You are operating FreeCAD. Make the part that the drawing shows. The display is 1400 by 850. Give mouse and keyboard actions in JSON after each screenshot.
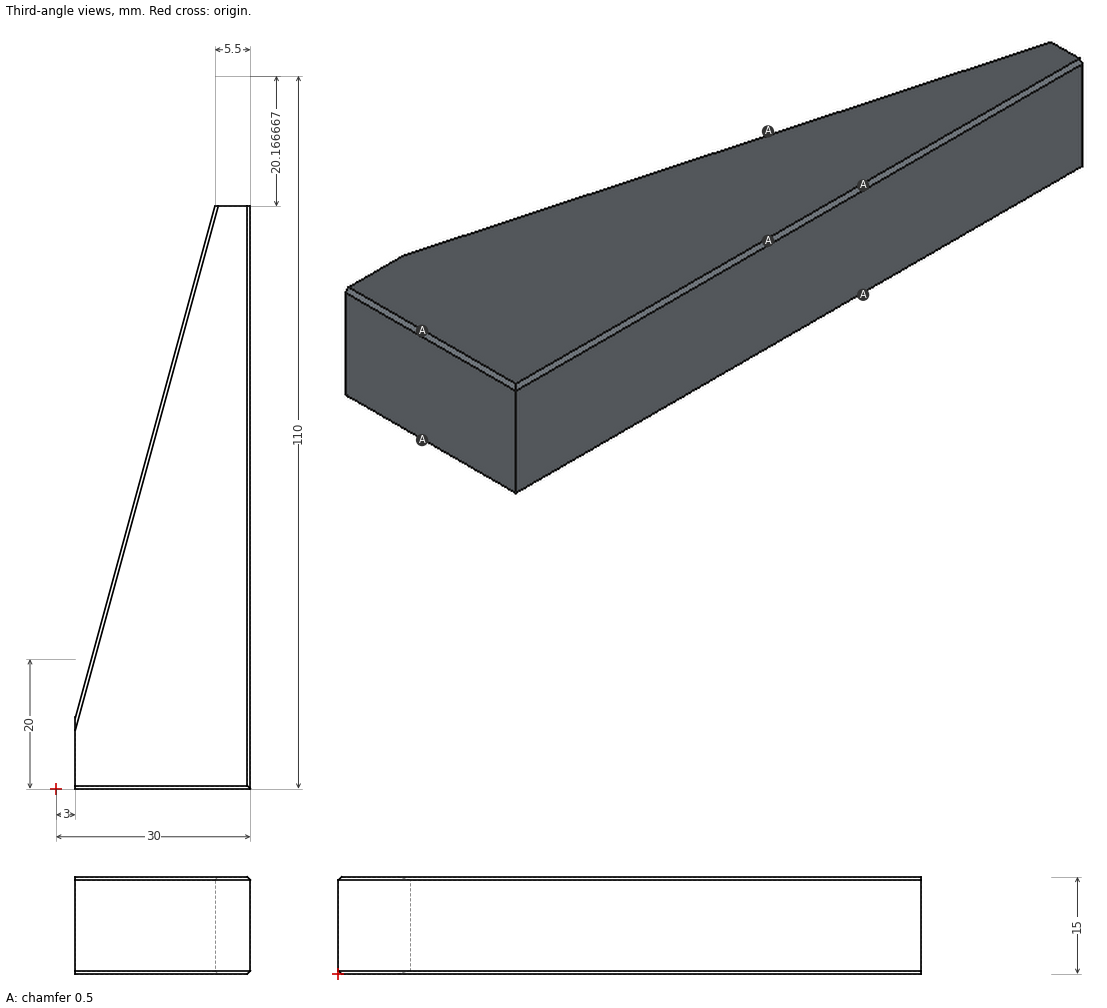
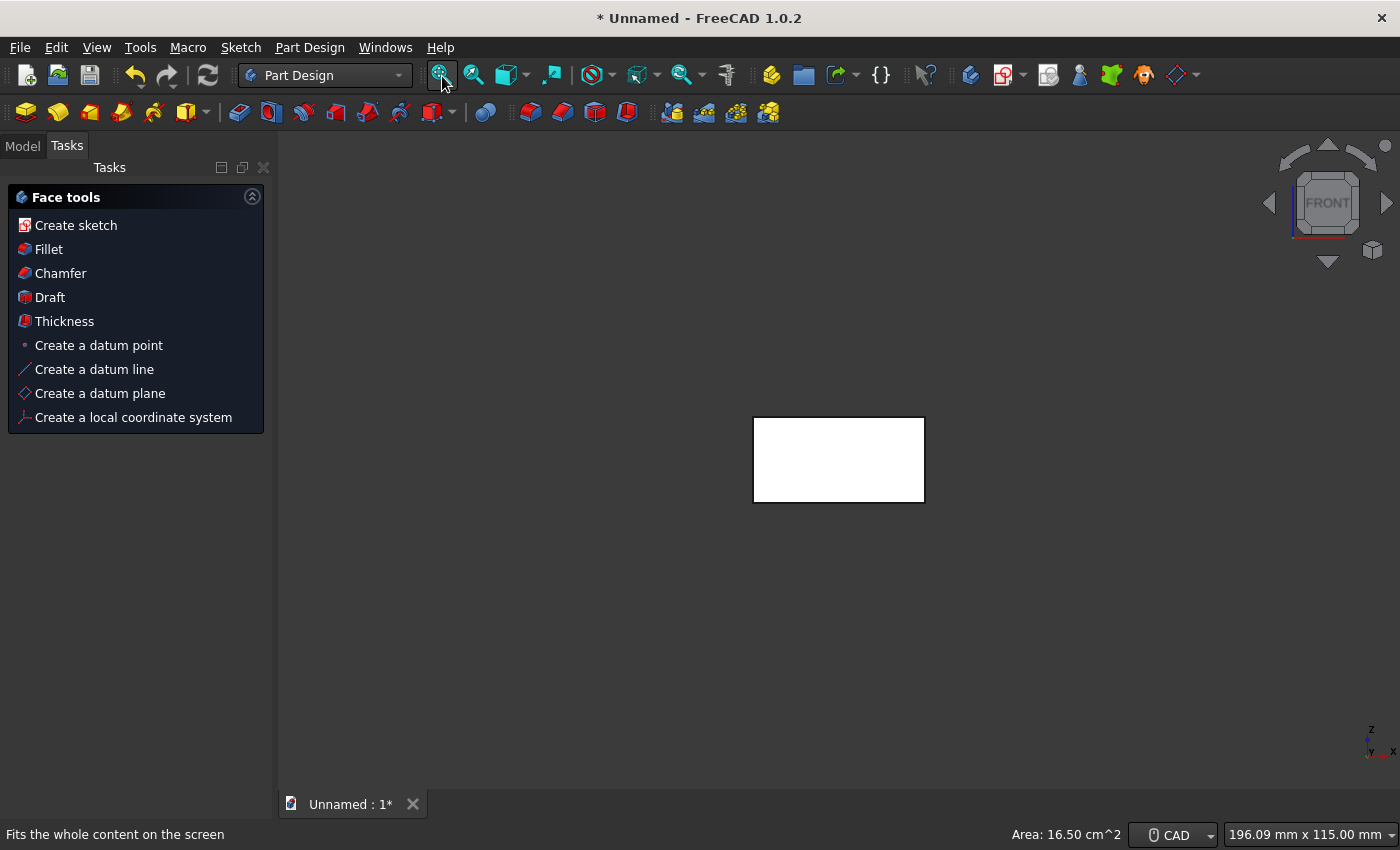
{"action": "key", "text": "3"}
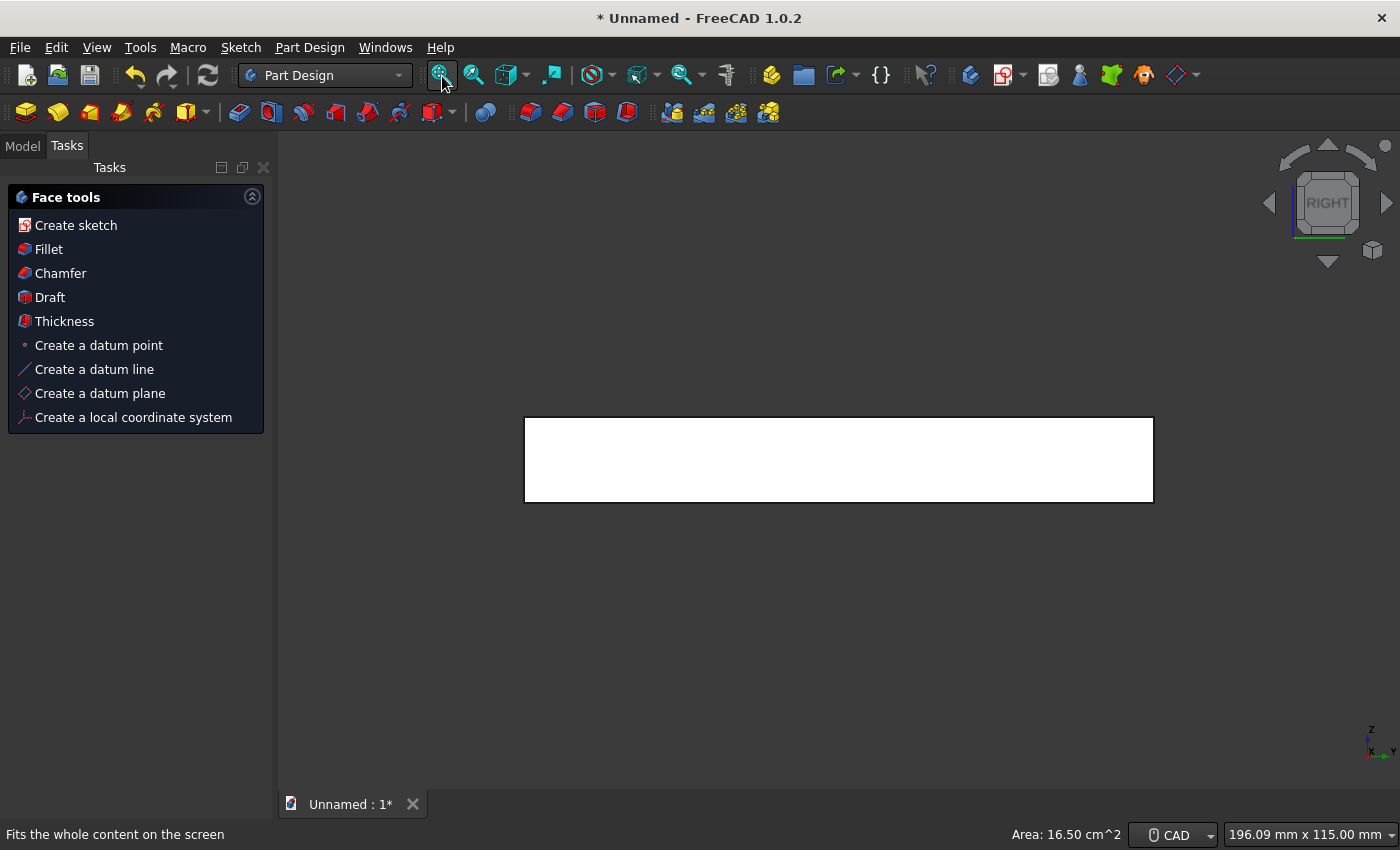
{"action": "key", "text": "5"}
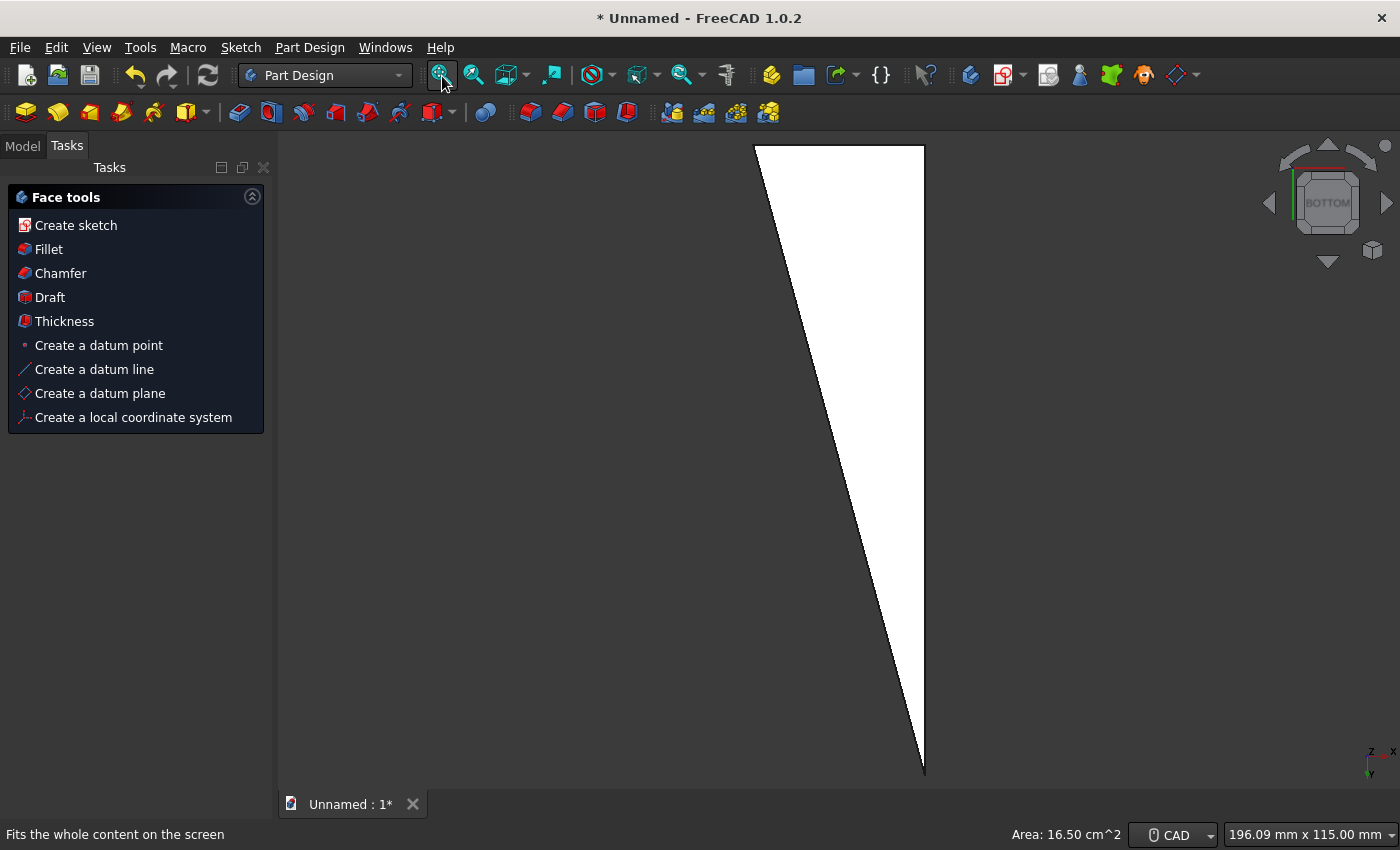
{"action": "left_click", "coordinate": [864, 279], "text": "ctrl"}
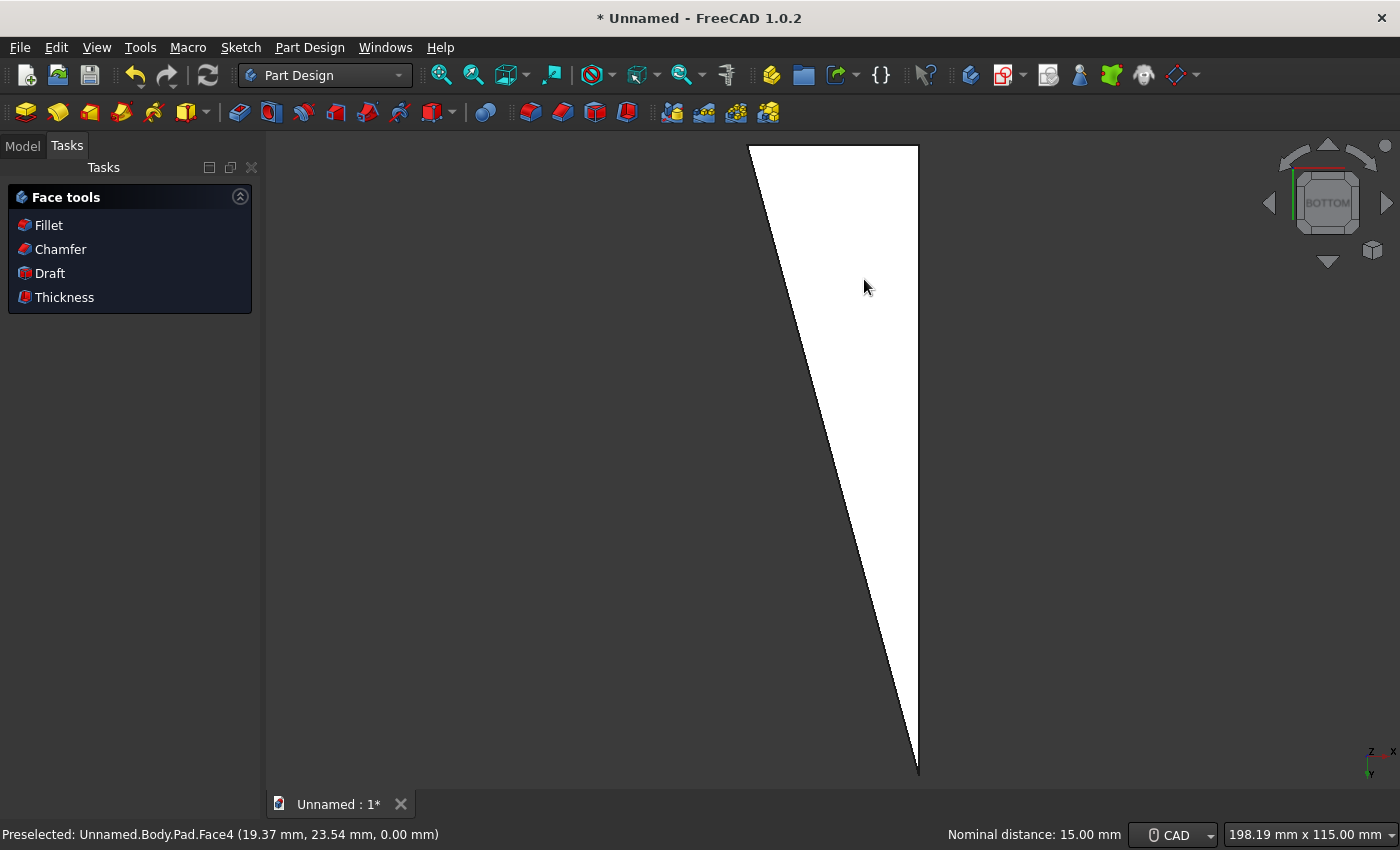
{"action": "left_click", "coordinate": [564, 112]}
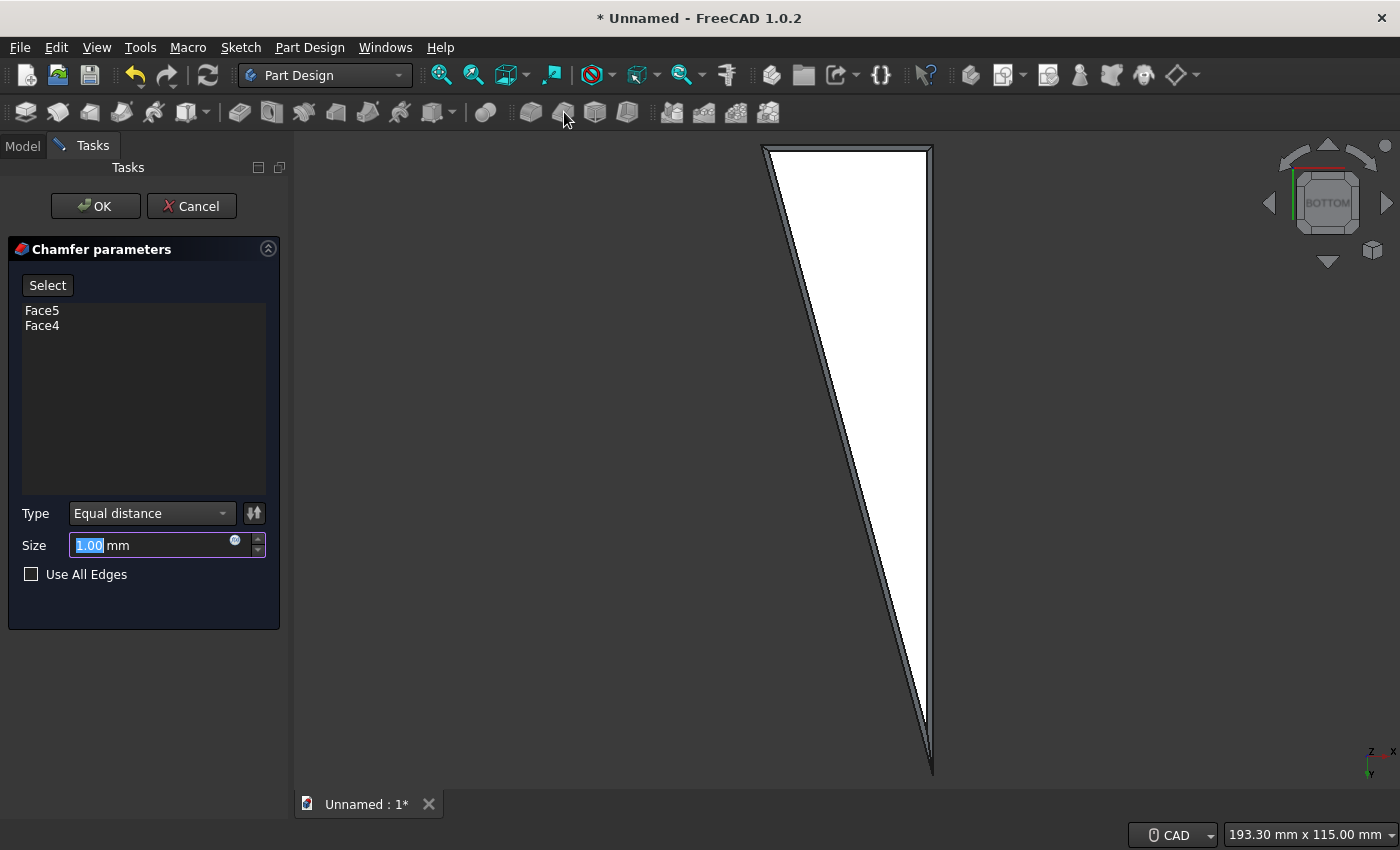
{"action": "type", "text": "0.5"}
{"action": "key", "text": "Tab"}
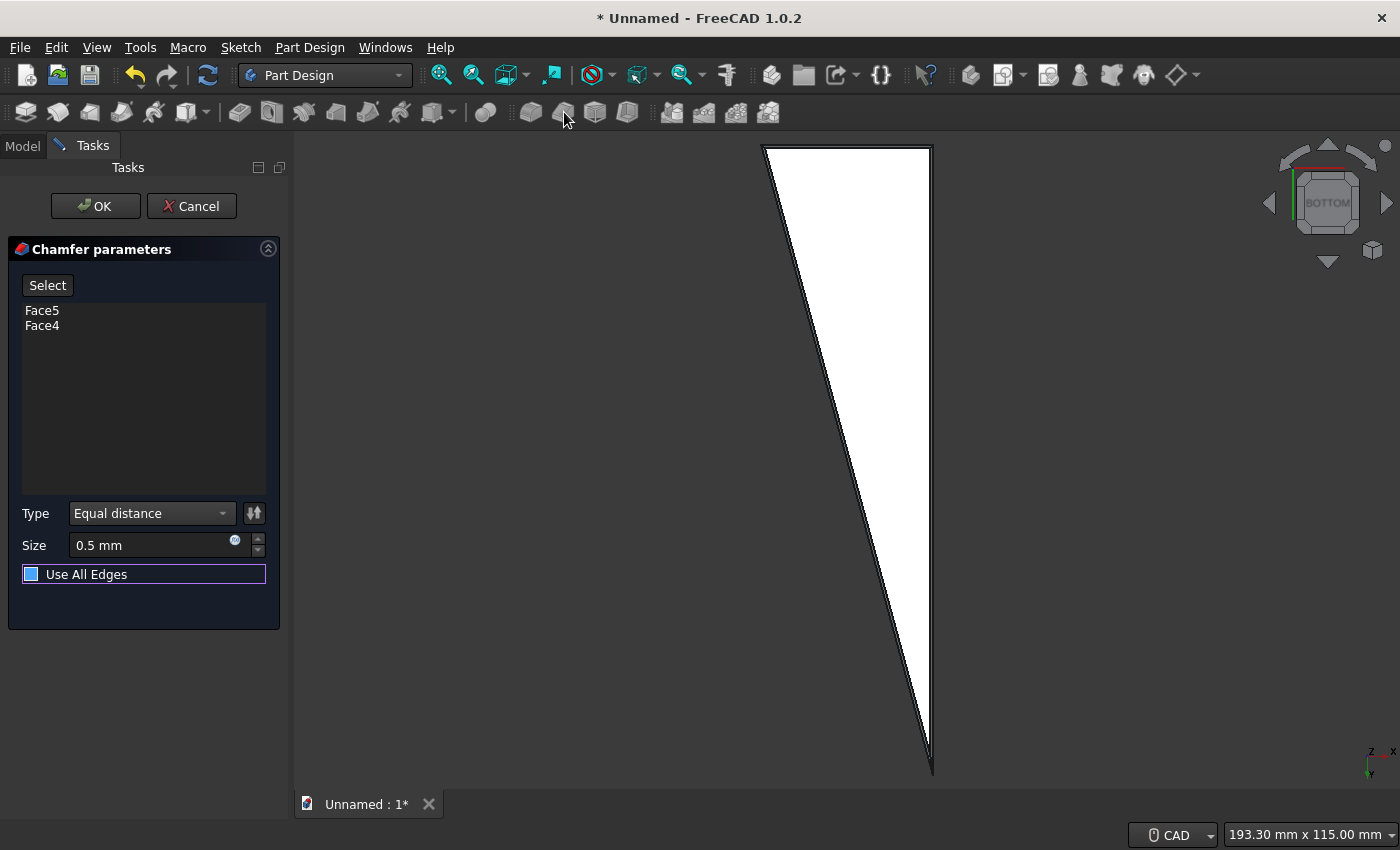
{"action": "left_click", "coordinate": [96, 206]}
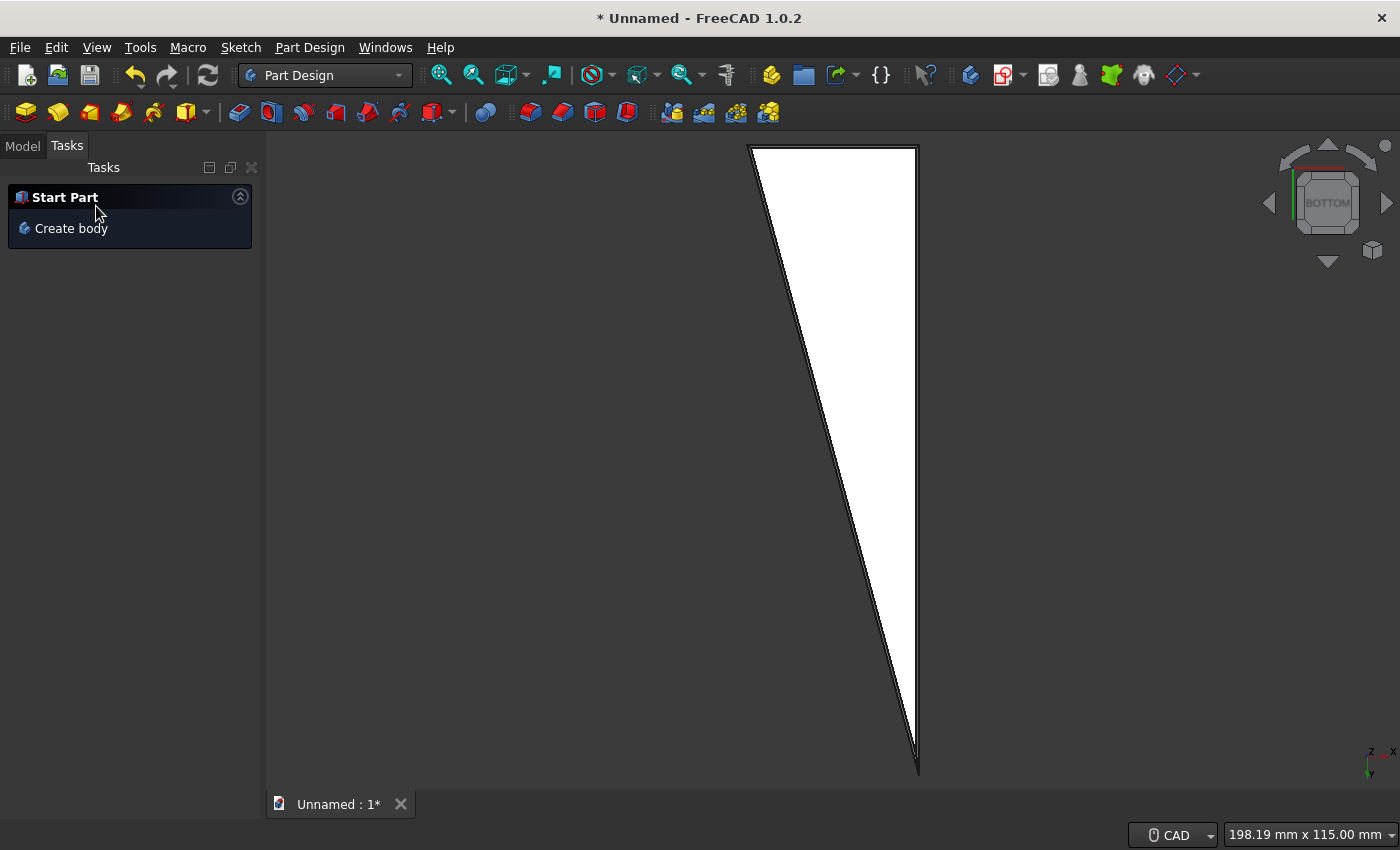
{"action": "key", "text": "0"}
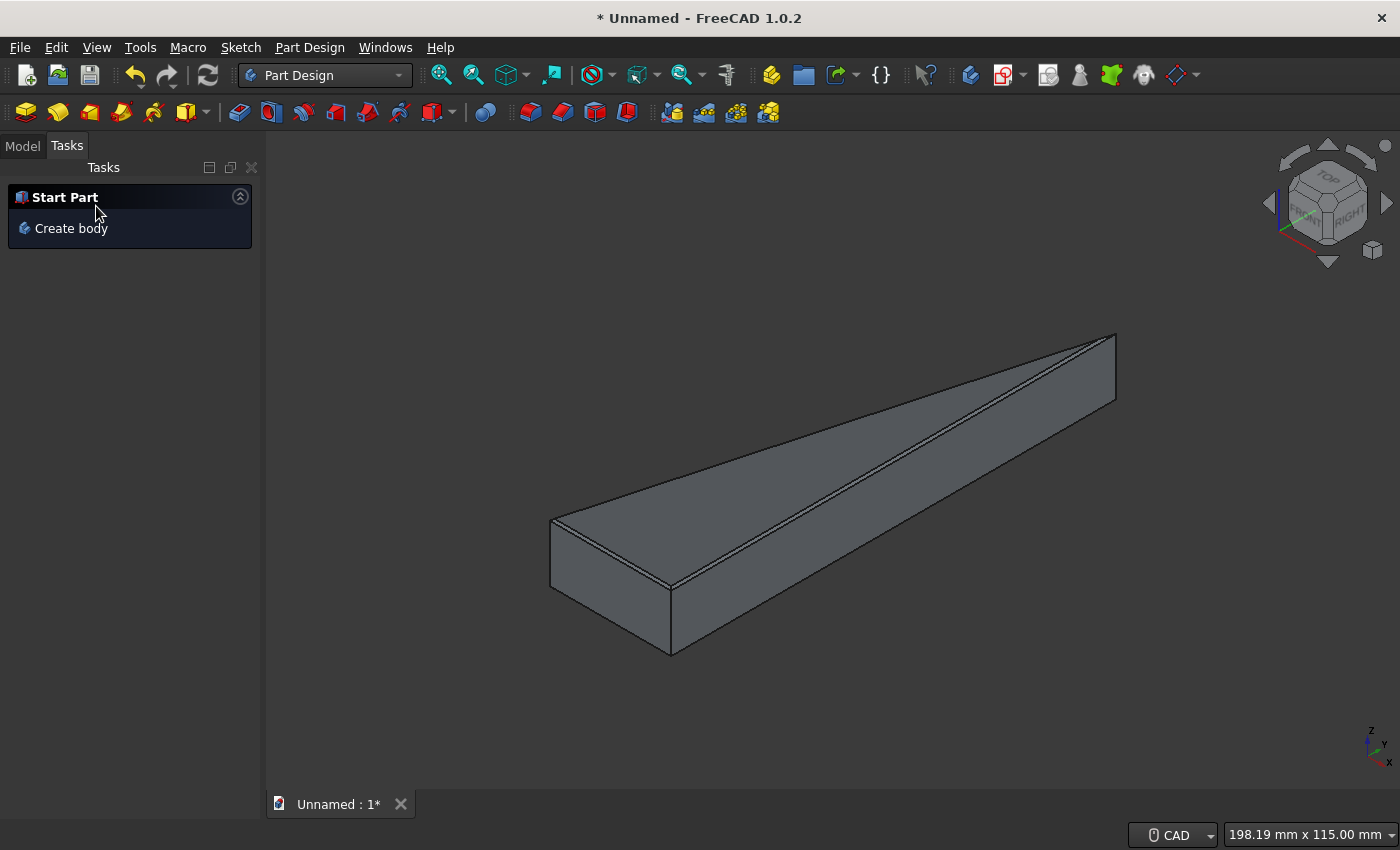
{"action": "left_click", "coordinate": [721, 508]}